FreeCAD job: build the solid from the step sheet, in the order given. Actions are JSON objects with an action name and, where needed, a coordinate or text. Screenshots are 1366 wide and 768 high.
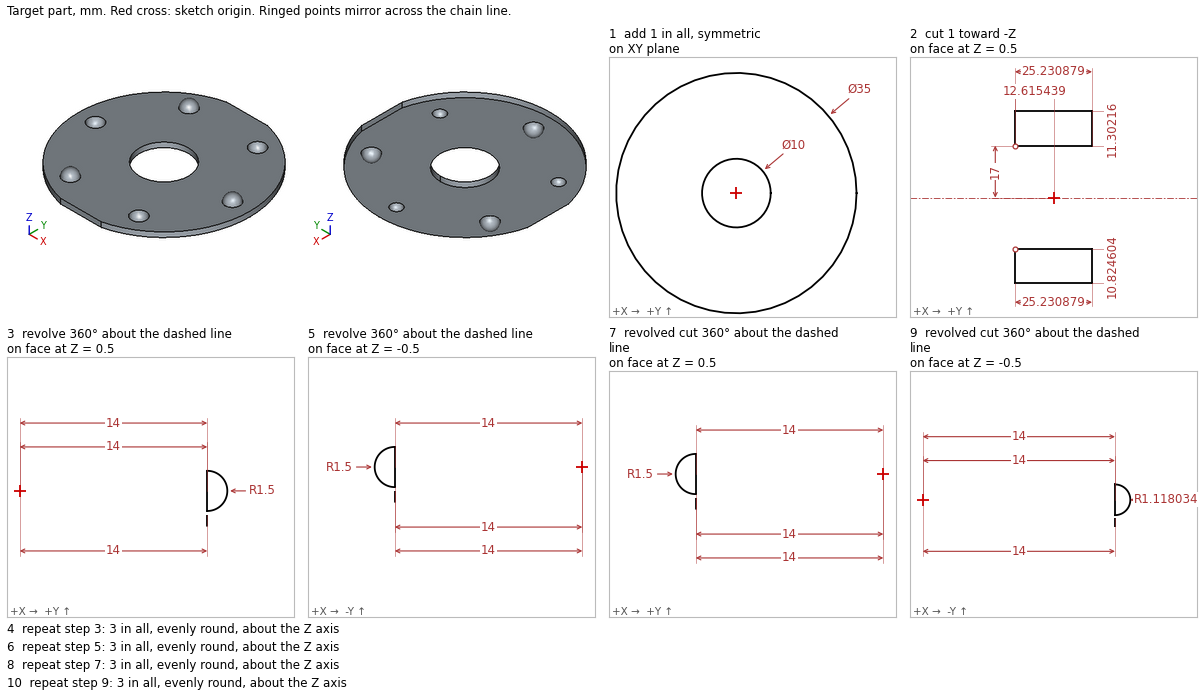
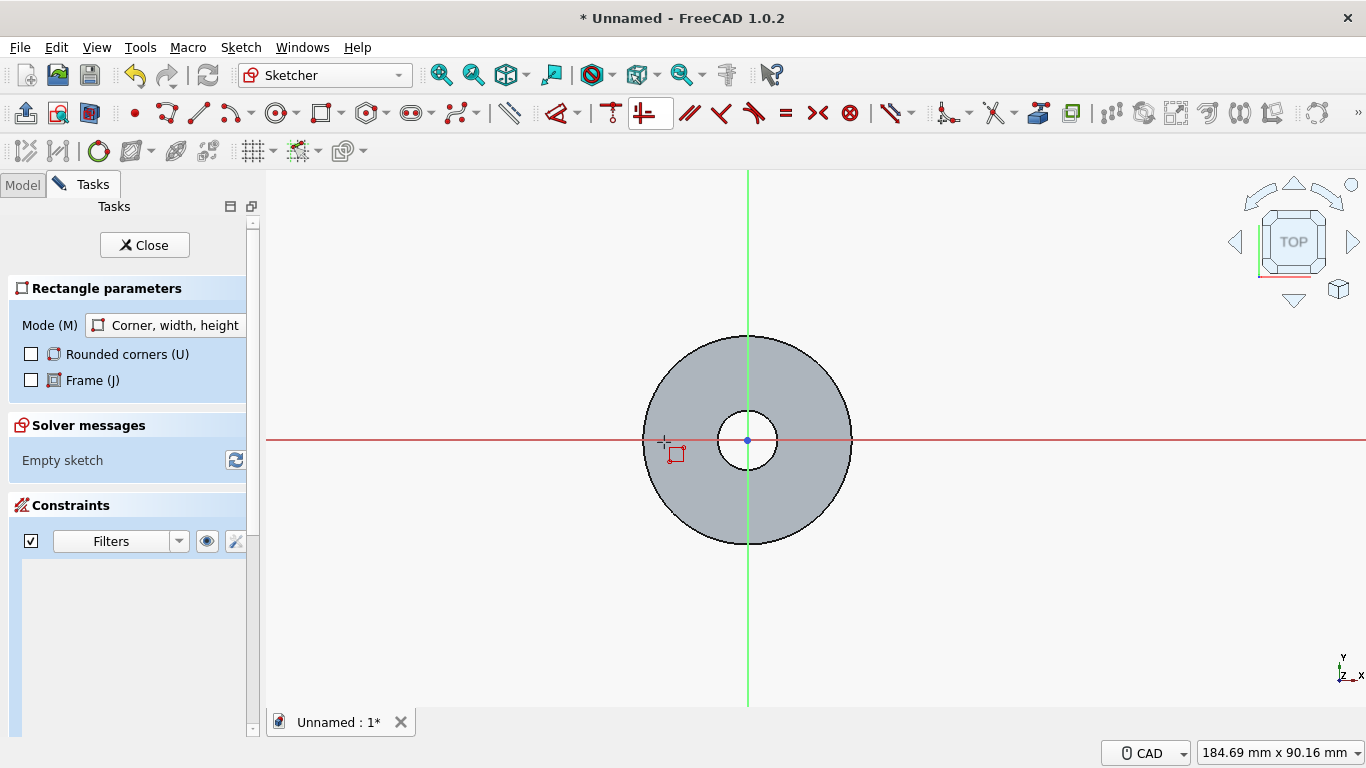
{"action": "left_click", "coordinate": [672, 272]}
{"action": "mouse_move", "coordinate": [823, 339]}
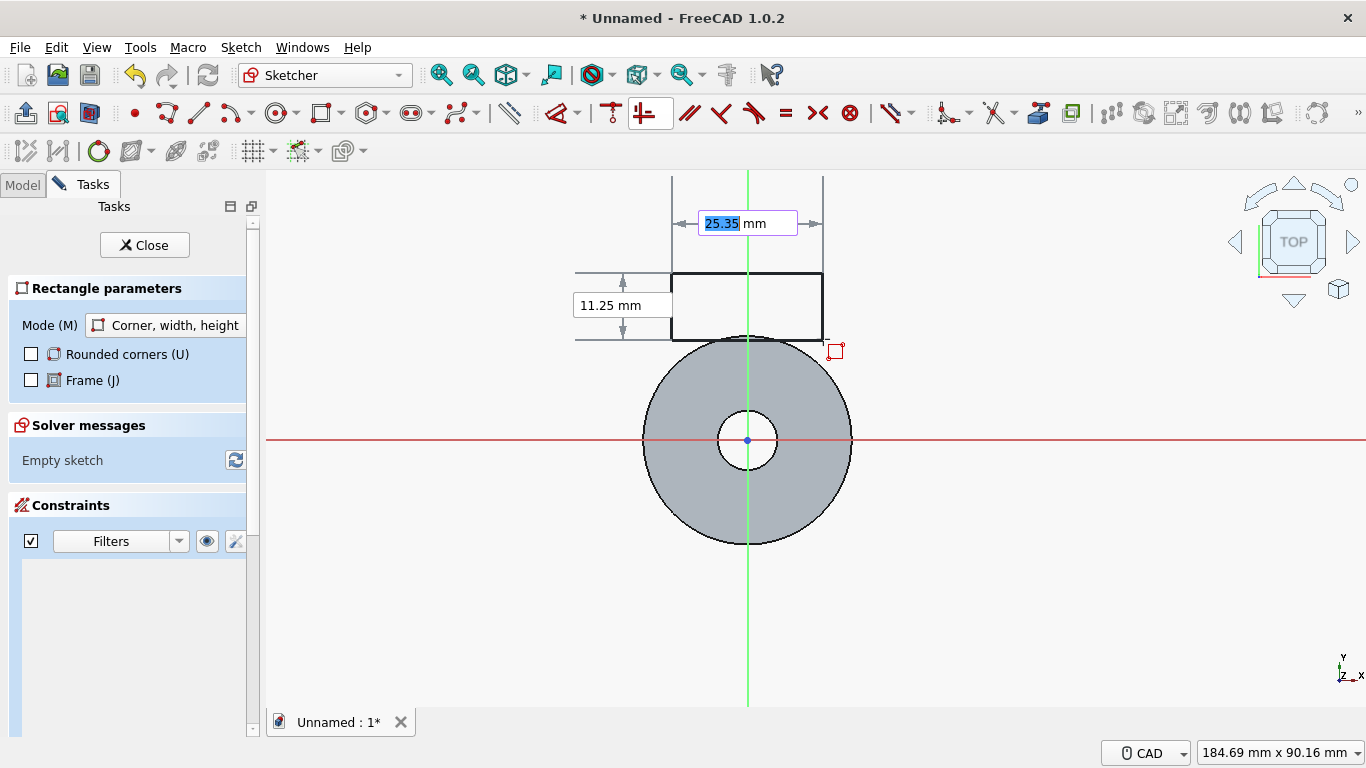
{"action": "type", "text": "25.230879"}
{"action": "key", "text": "Tab"}
{"action": "type", "text": "11.30216"}
{"action": "key", "text": "Return"}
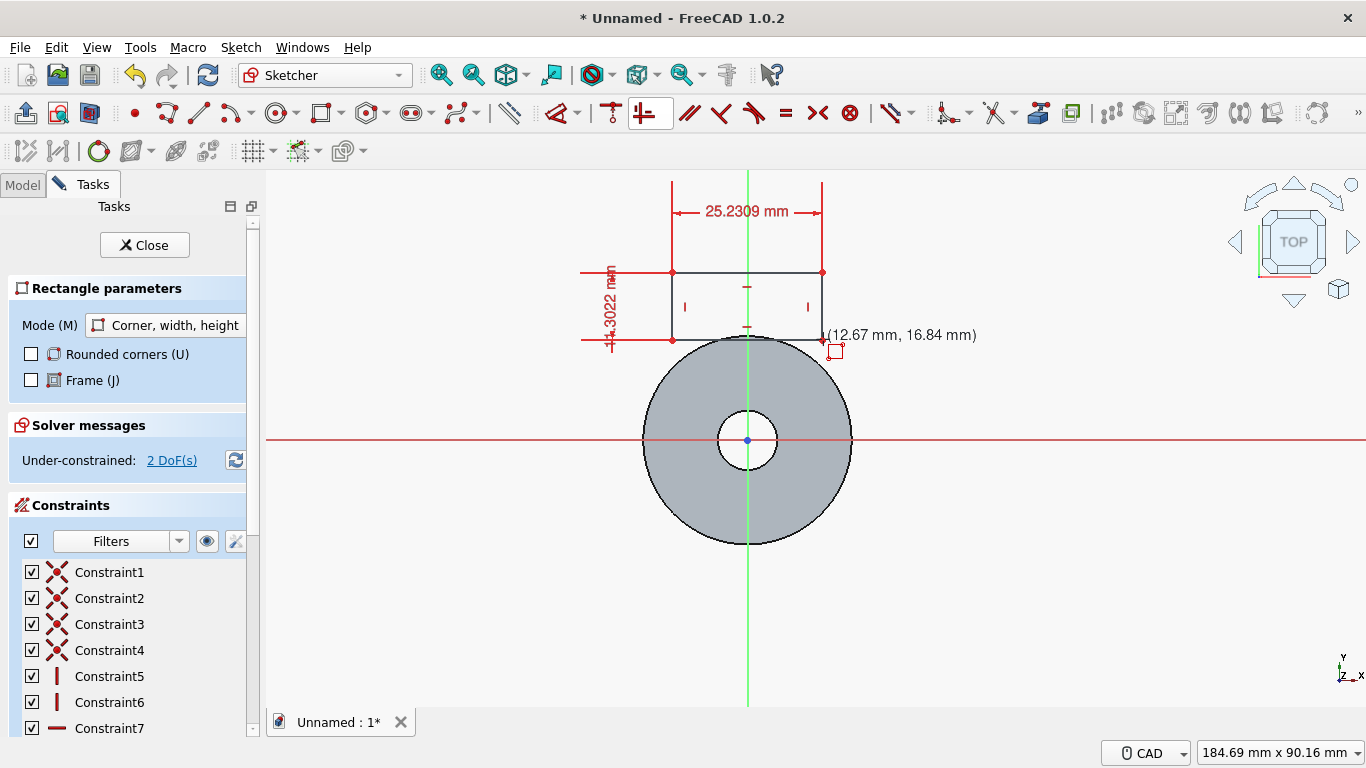
{"action": "left_click", "coordinate": [672, 542]}
{"action": "mouse_move", "coordinate": [823, 606]}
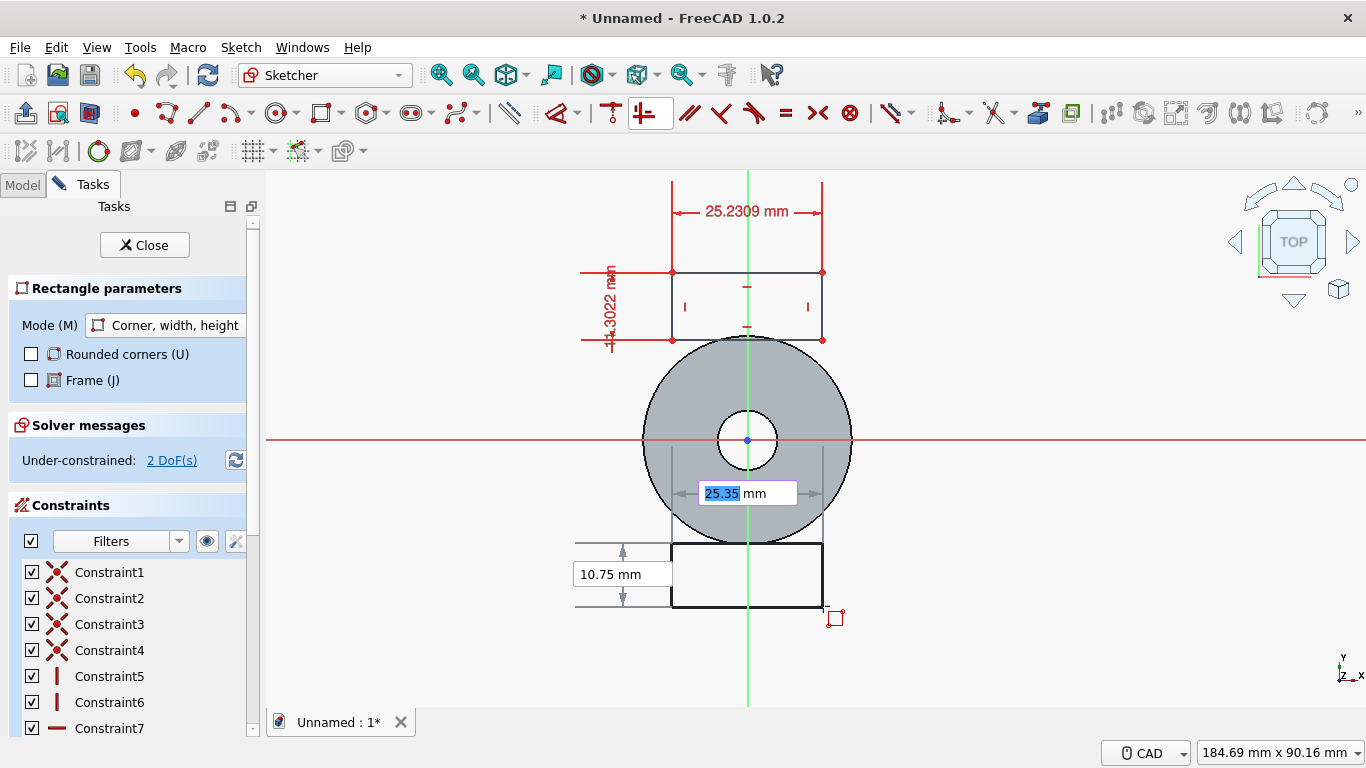
{"action": "type", "text": "25.230879"}
{"action": "key", "text": "Tab"}
{"action": "type", "text": "10.824604"}
{"action": "key", "text": "Return"}
{"action": "key", "text": "Escape"}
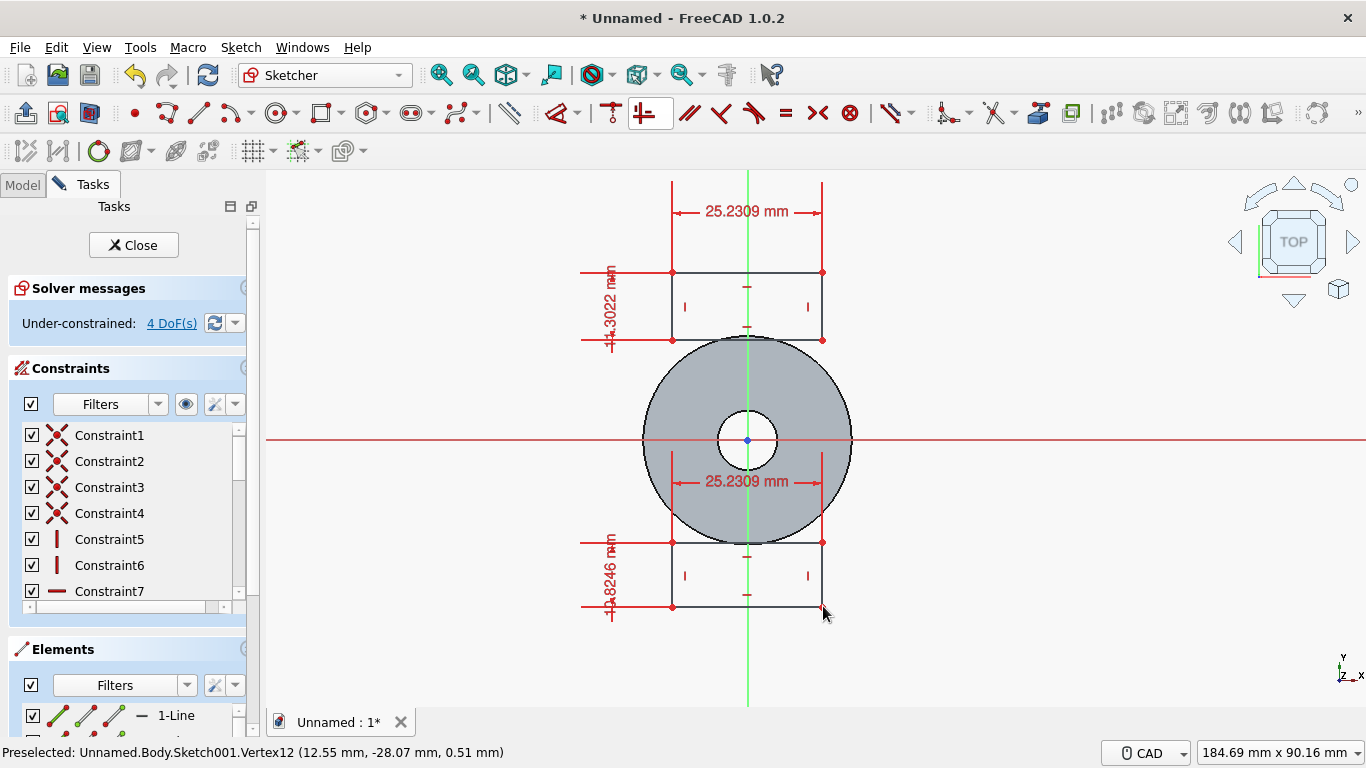
{"action": "left_click", "coordinate": [672, 340]}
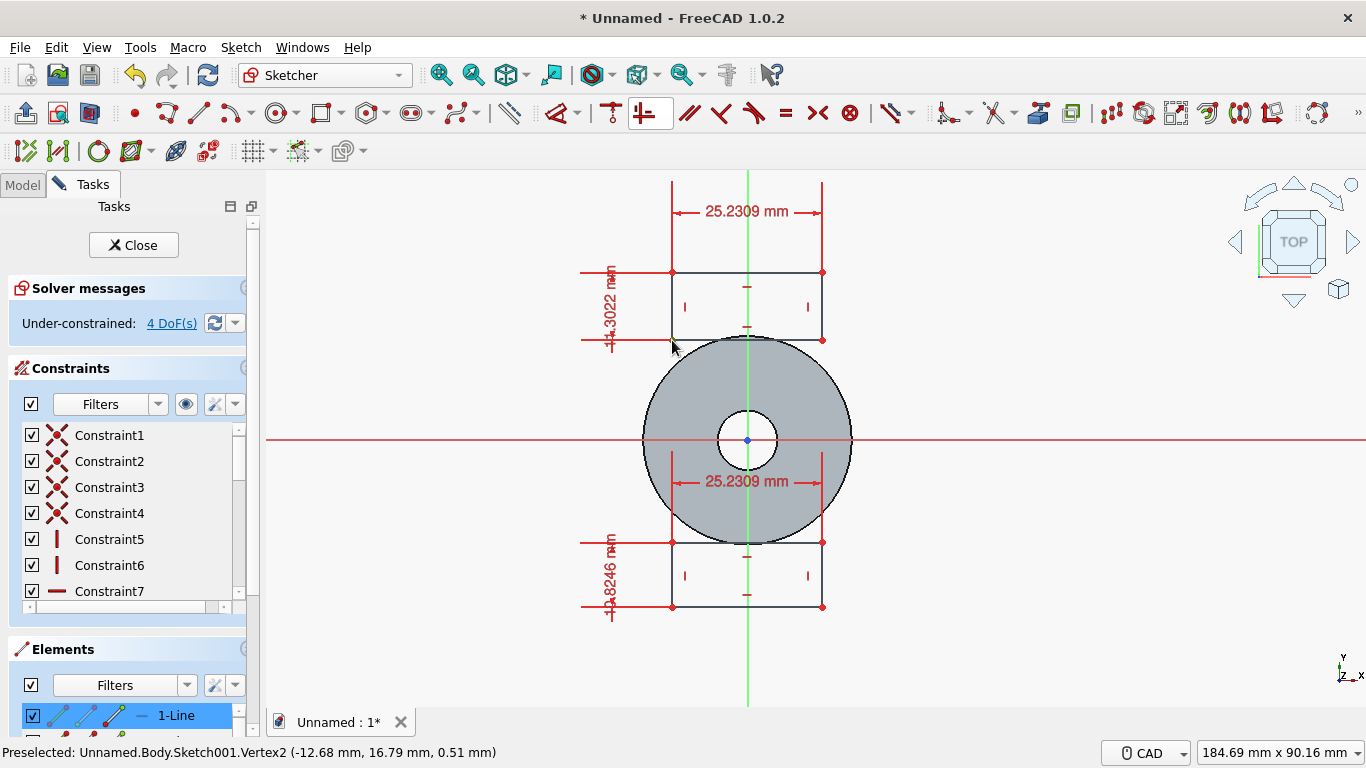
{"action": "left_click", "coordinate": [672, 543]}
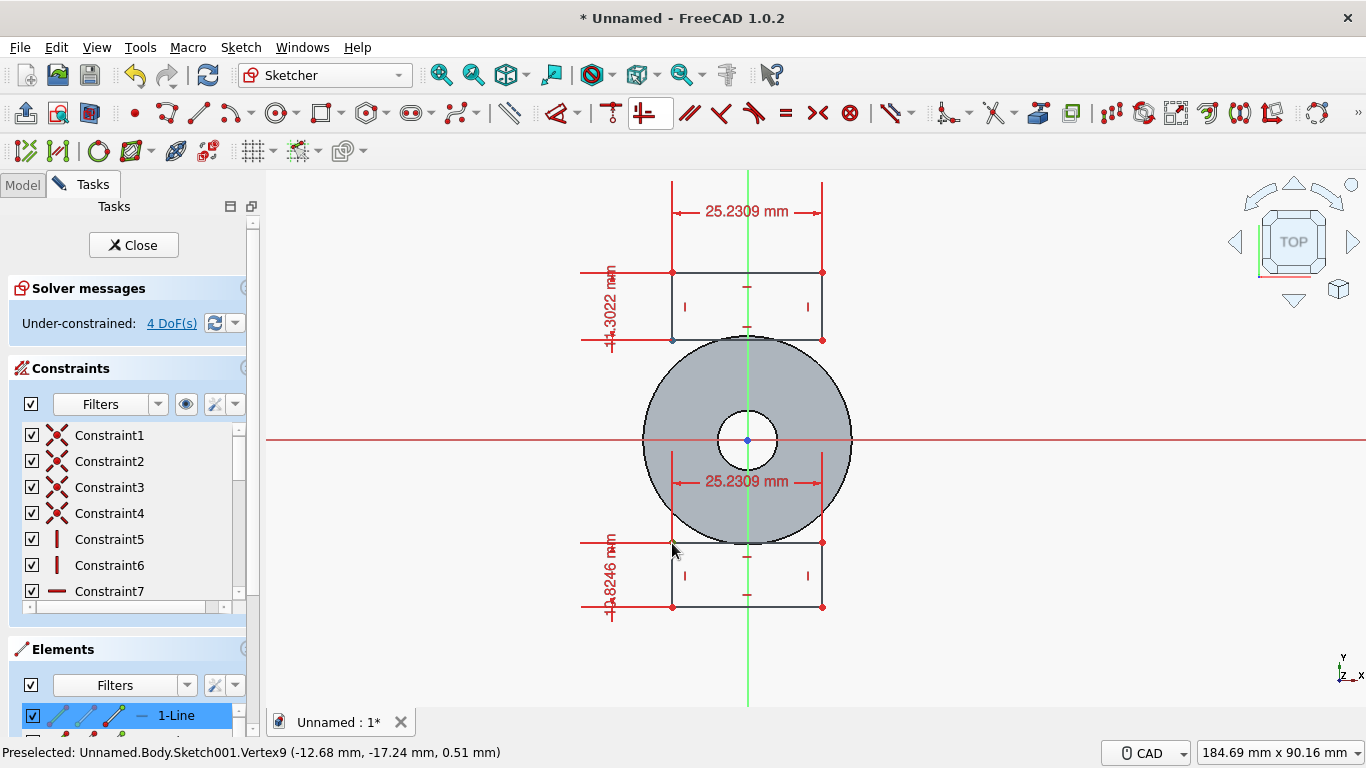
{"action": "left_click", "coordinate": [359, 440]}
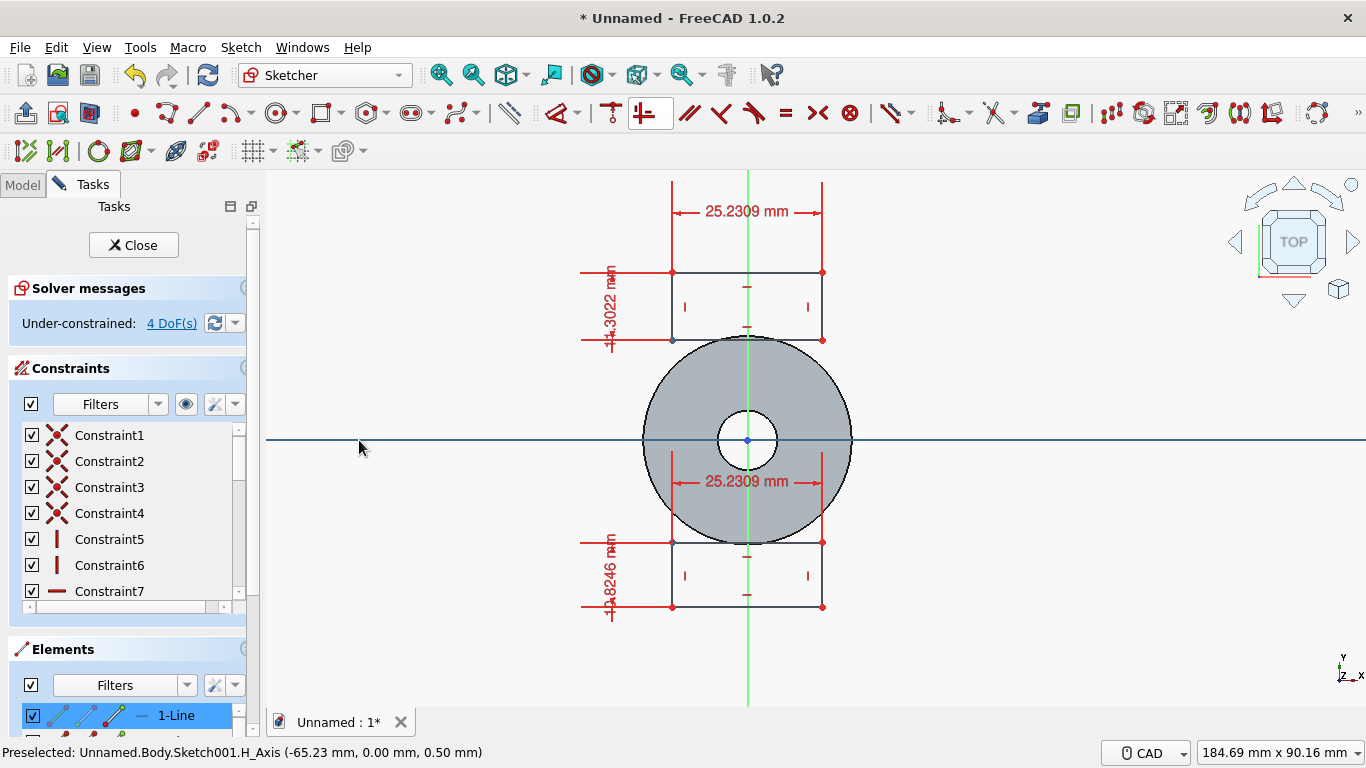
{"action": "left_click", "coordinate": [818, 114]}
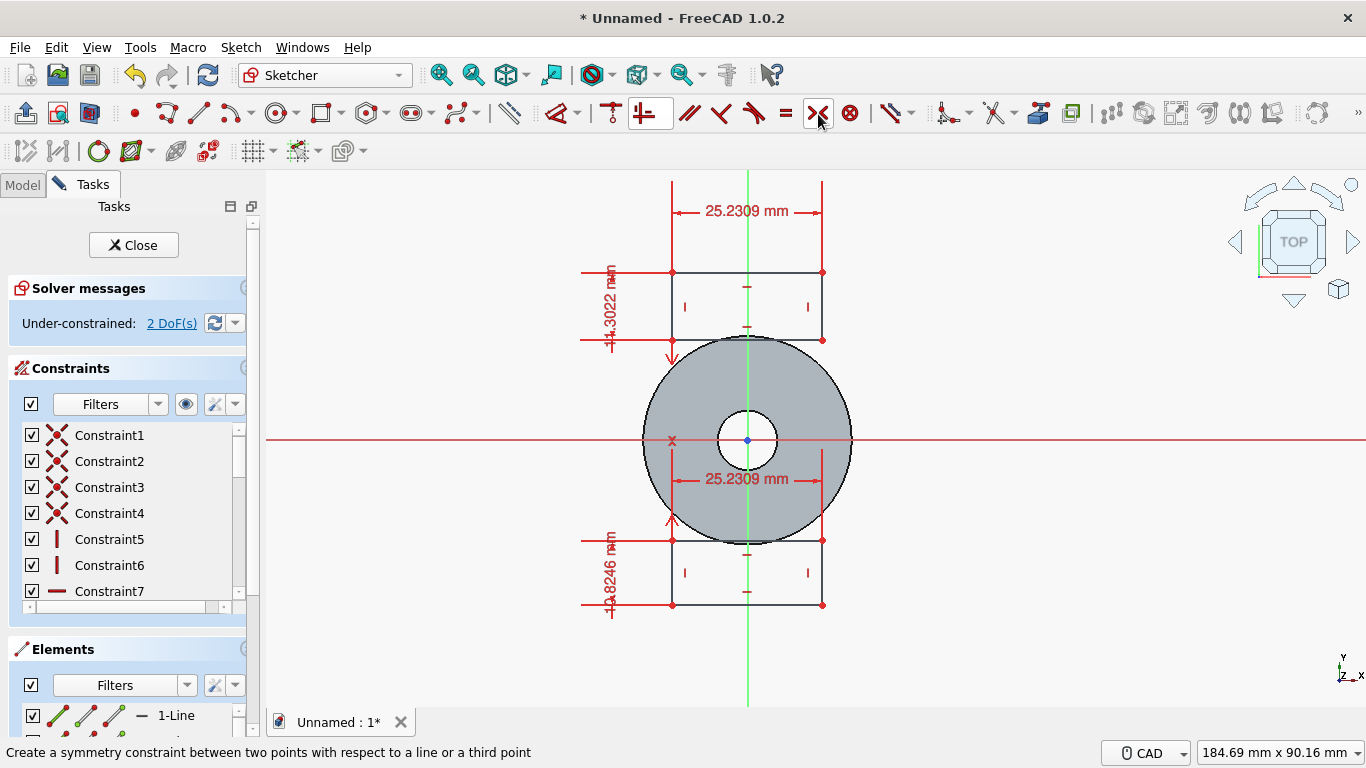
{"action": "key", "text": "d"}